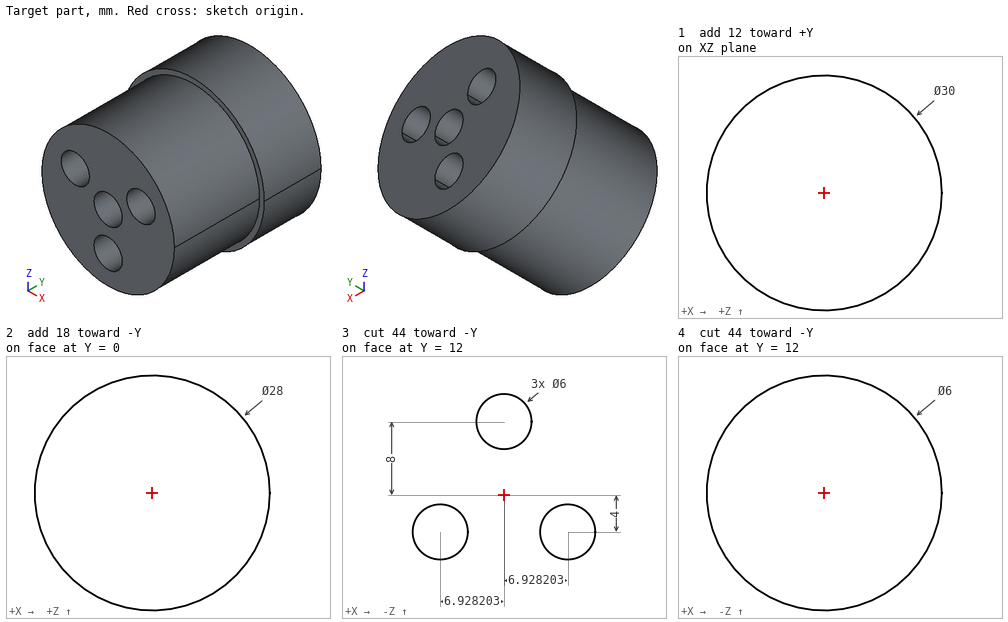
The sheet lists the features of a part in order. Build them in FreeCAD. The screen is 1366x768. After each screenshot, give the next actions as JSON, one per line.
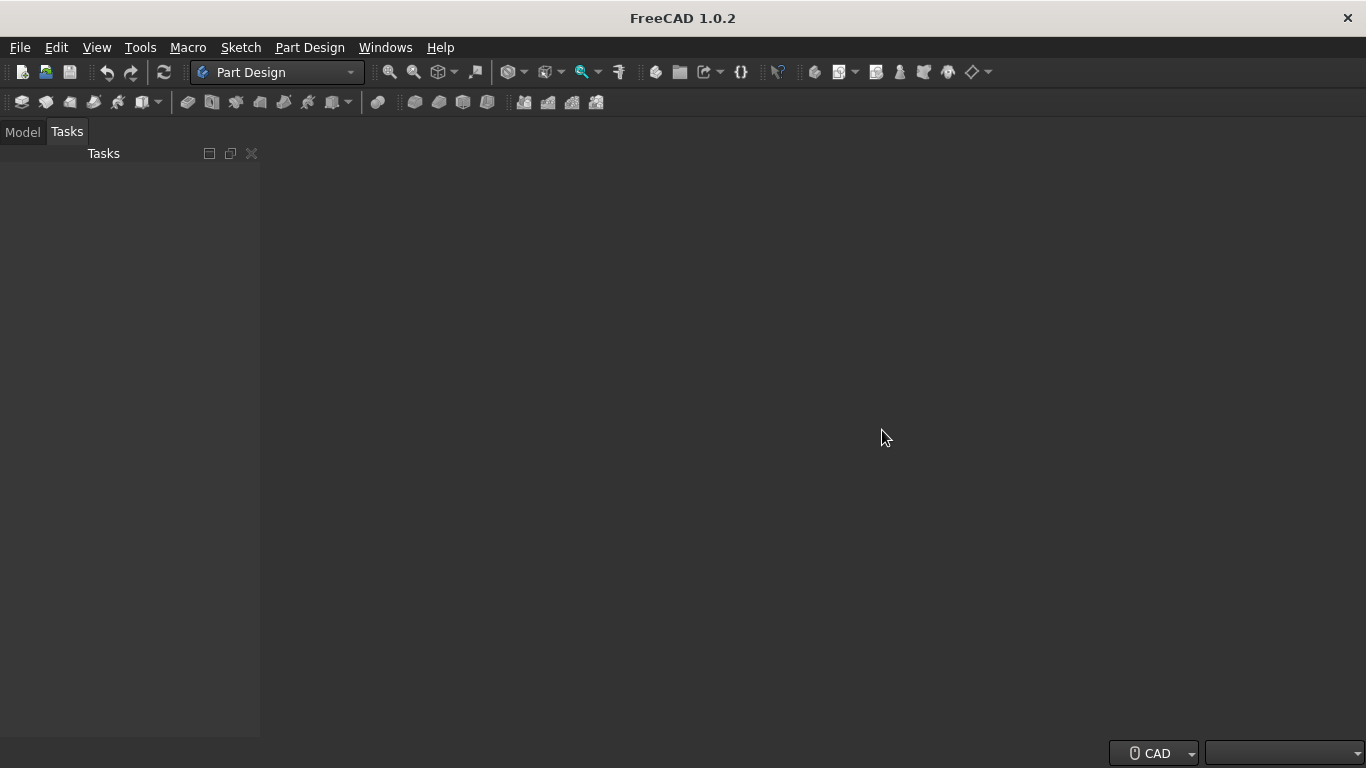
{"action": "left_click", "coordinate": [22, 72]}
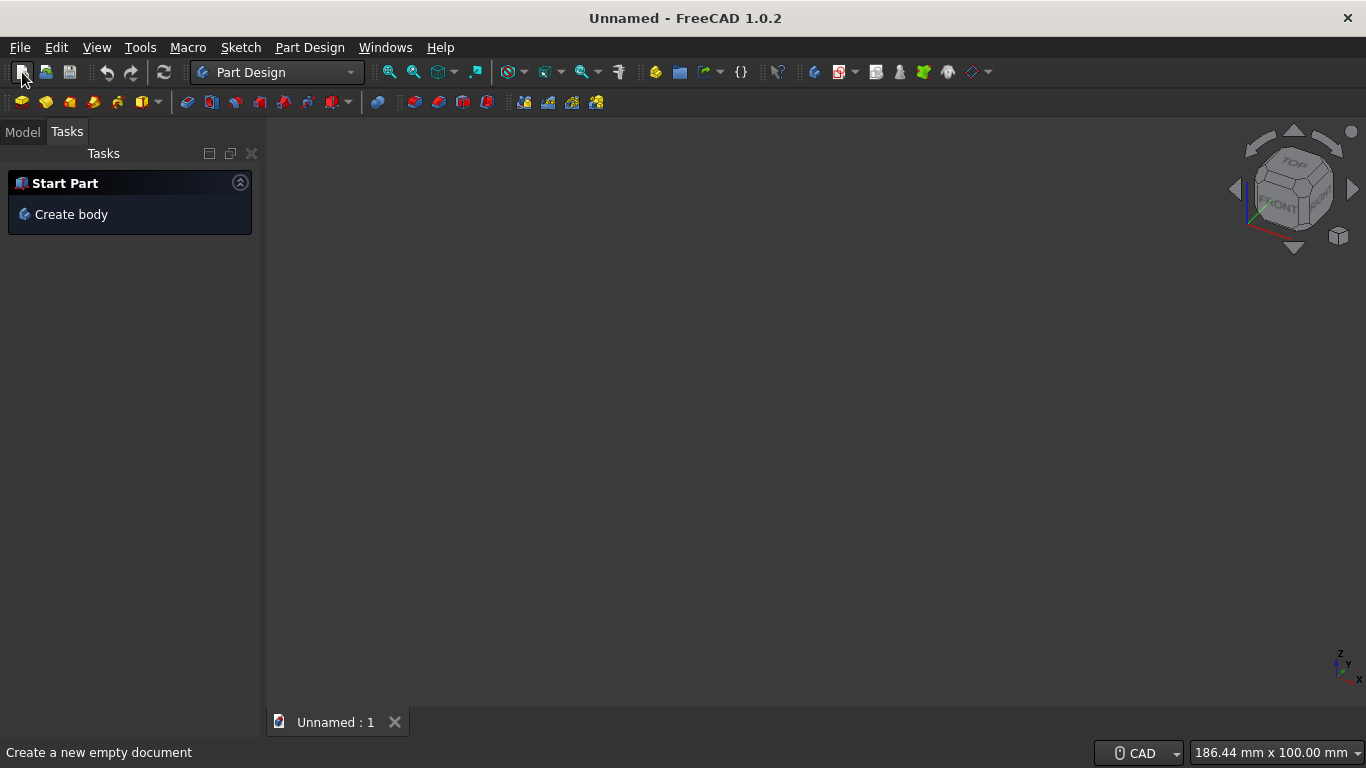
{"action": "left_click", "coordinate": [840, 72]}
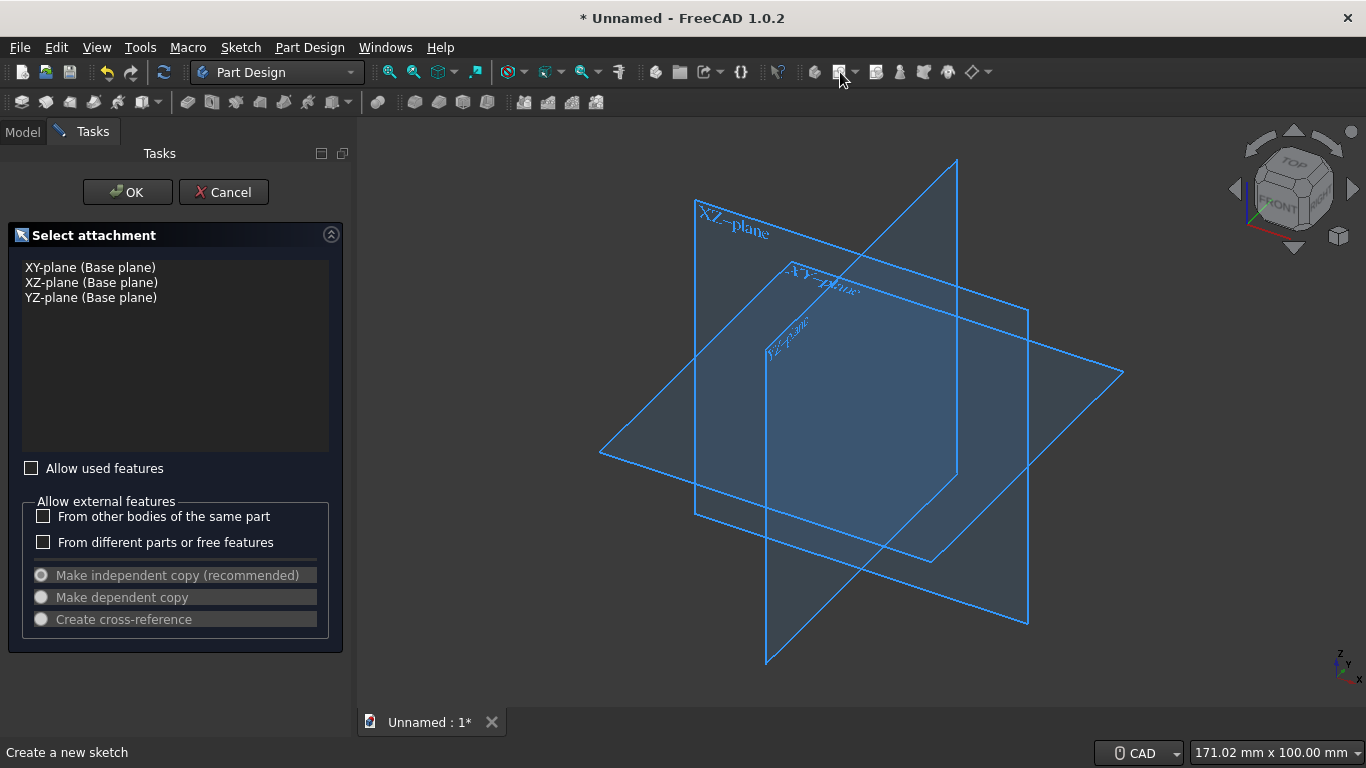
{"action": "left_click", "coordinate": [82, 282]}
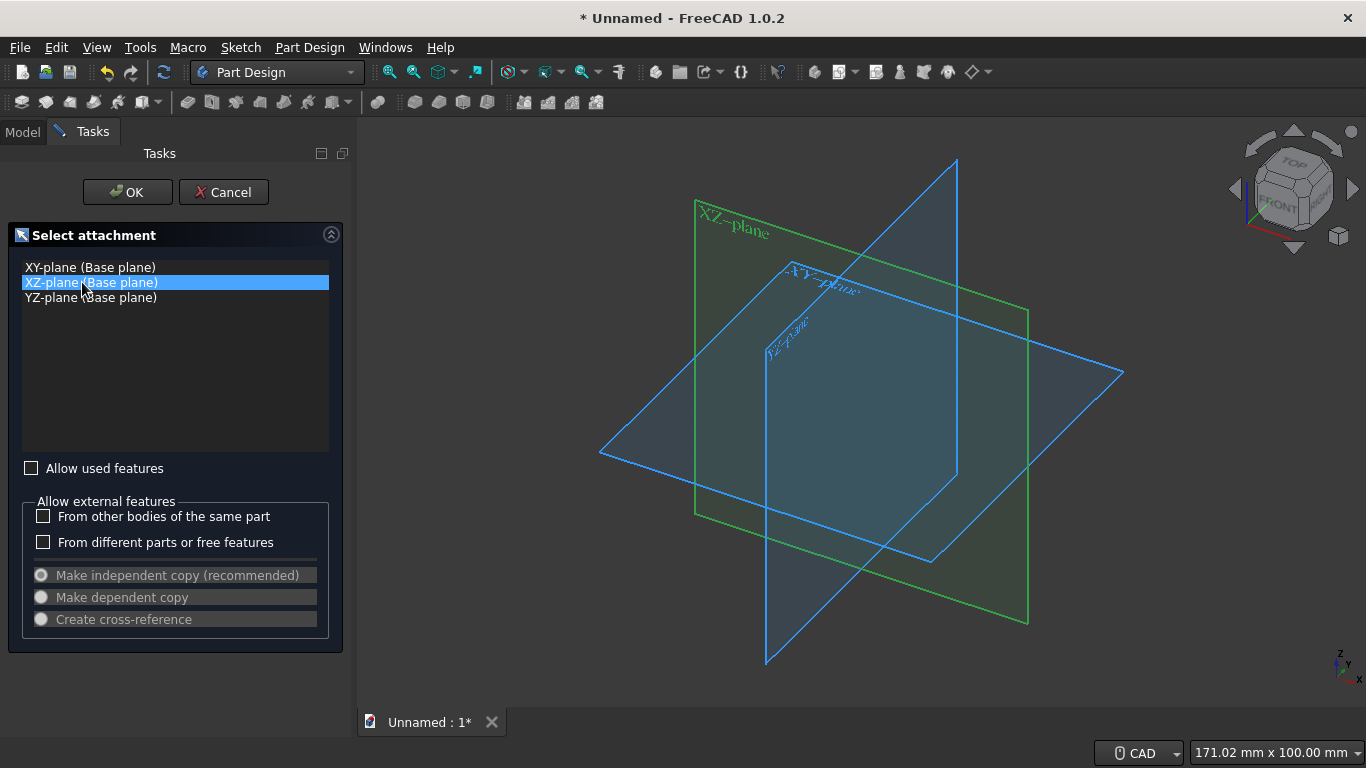
{"action": "left_click", "coordinate": [128, 192]}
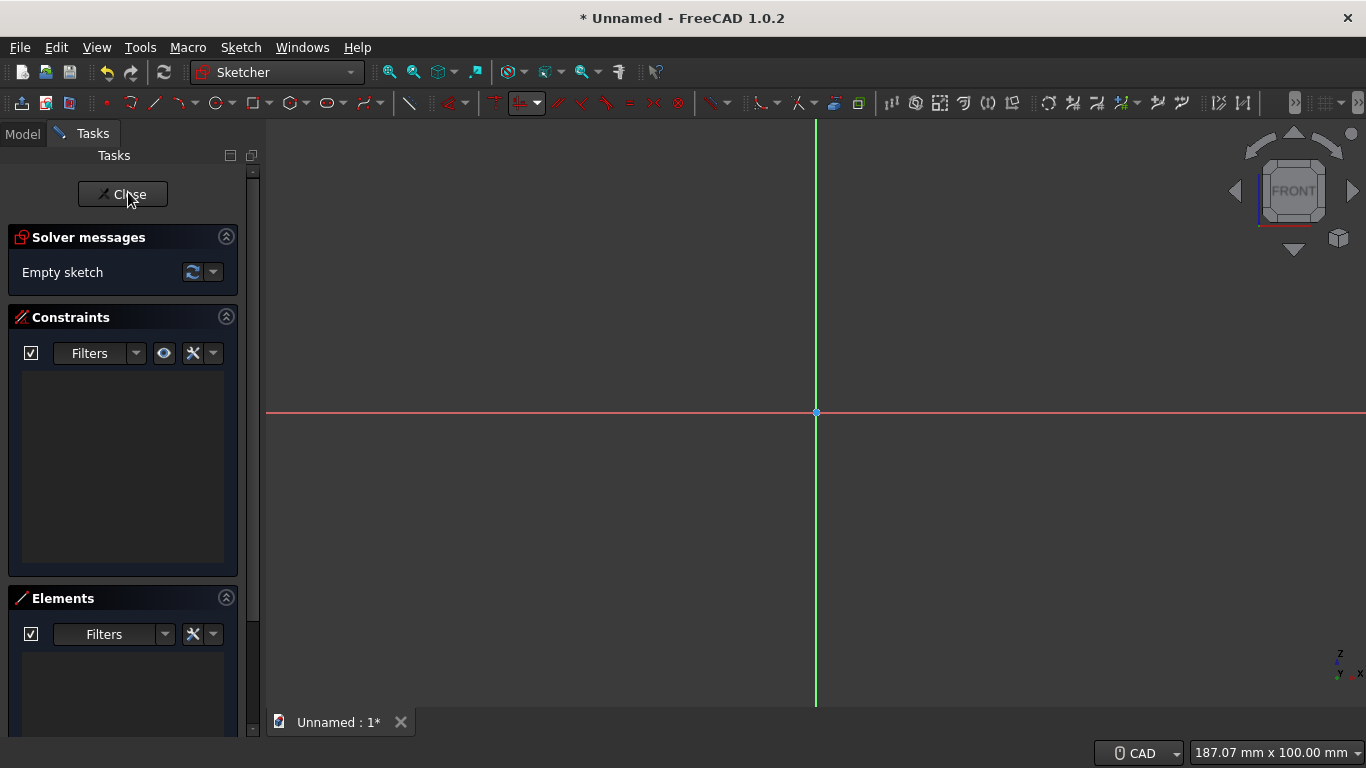
{"action": "scroll", "coordinate": [872, 413], "scroll_direction": "up", "scroll_amount": 4}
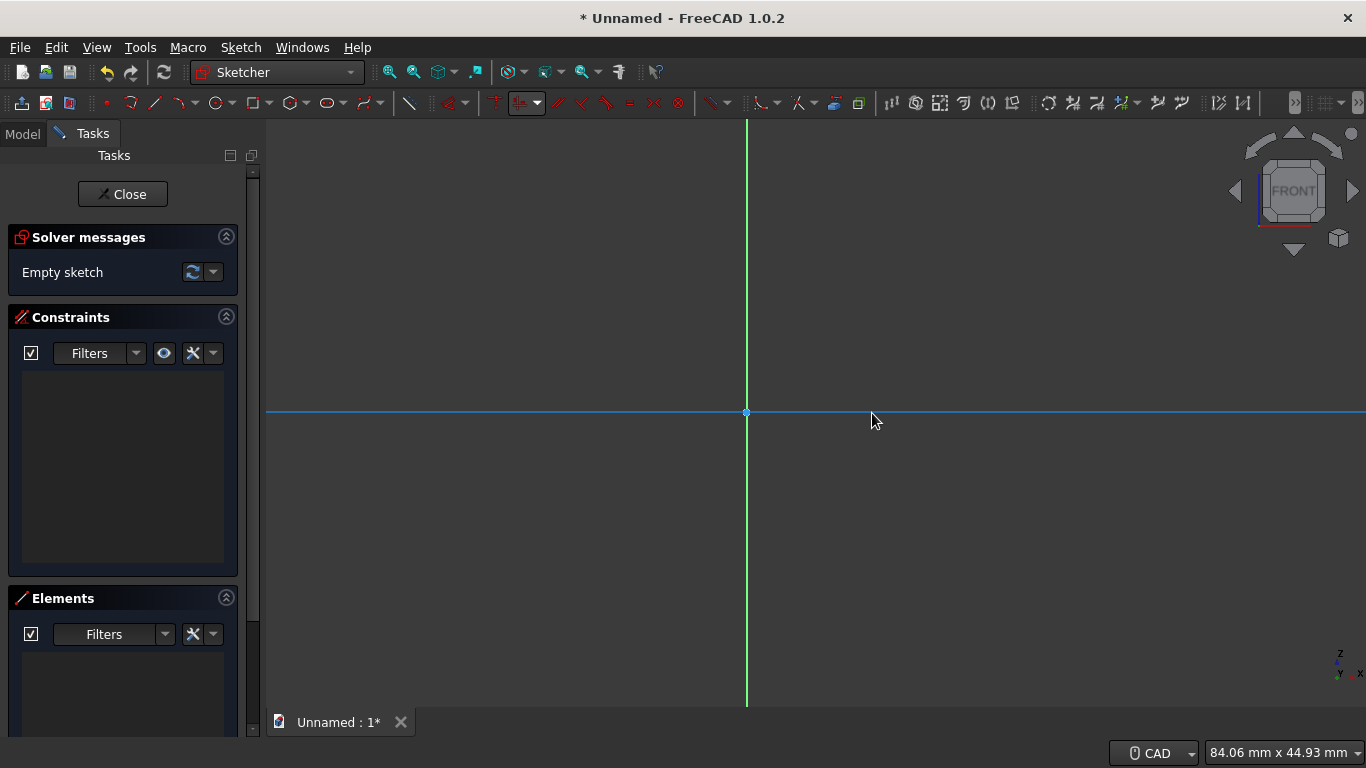
{"action": "left_click", "coordinate": [216, 104]}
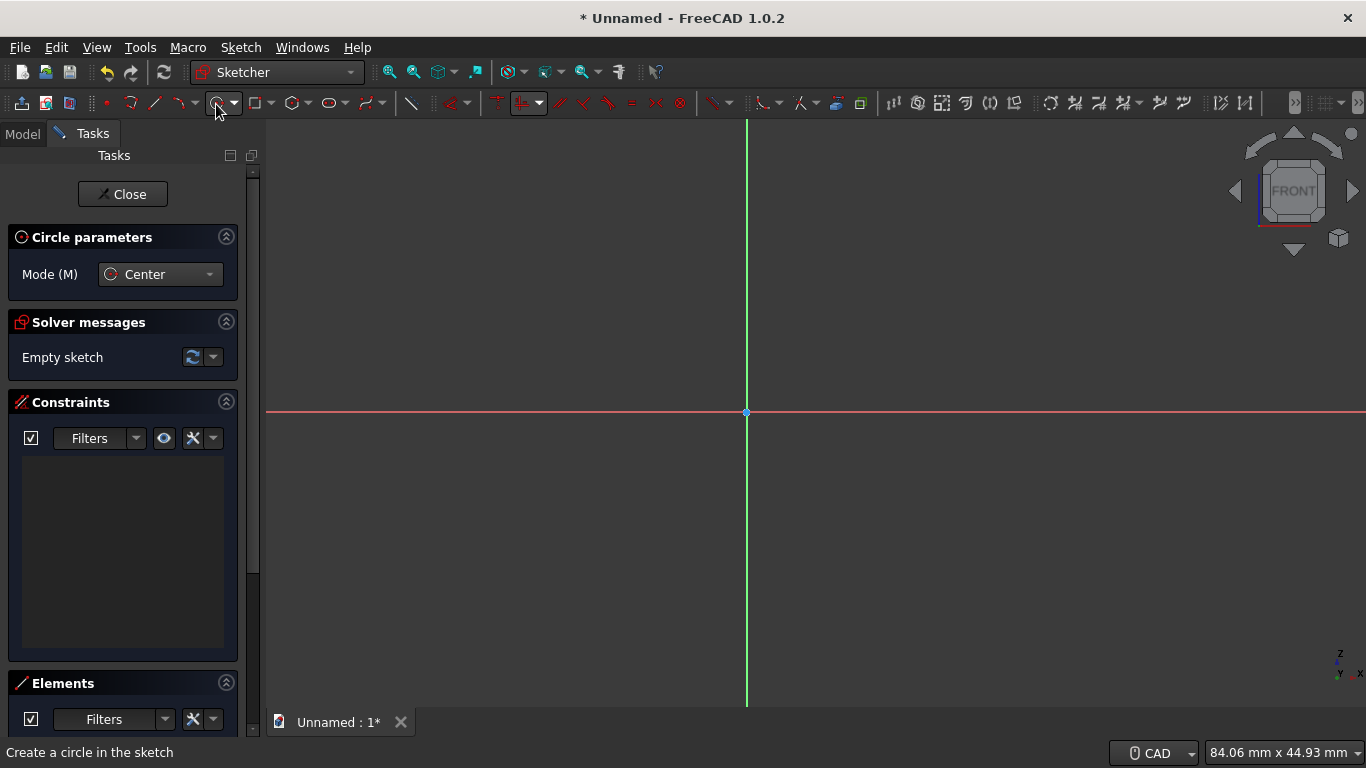
{"action": "left_click", "coordinate": [747, 412]}
{"action": "left_click", "coordinate": [885, 274]}
{"action": "key", "text": "Escape"}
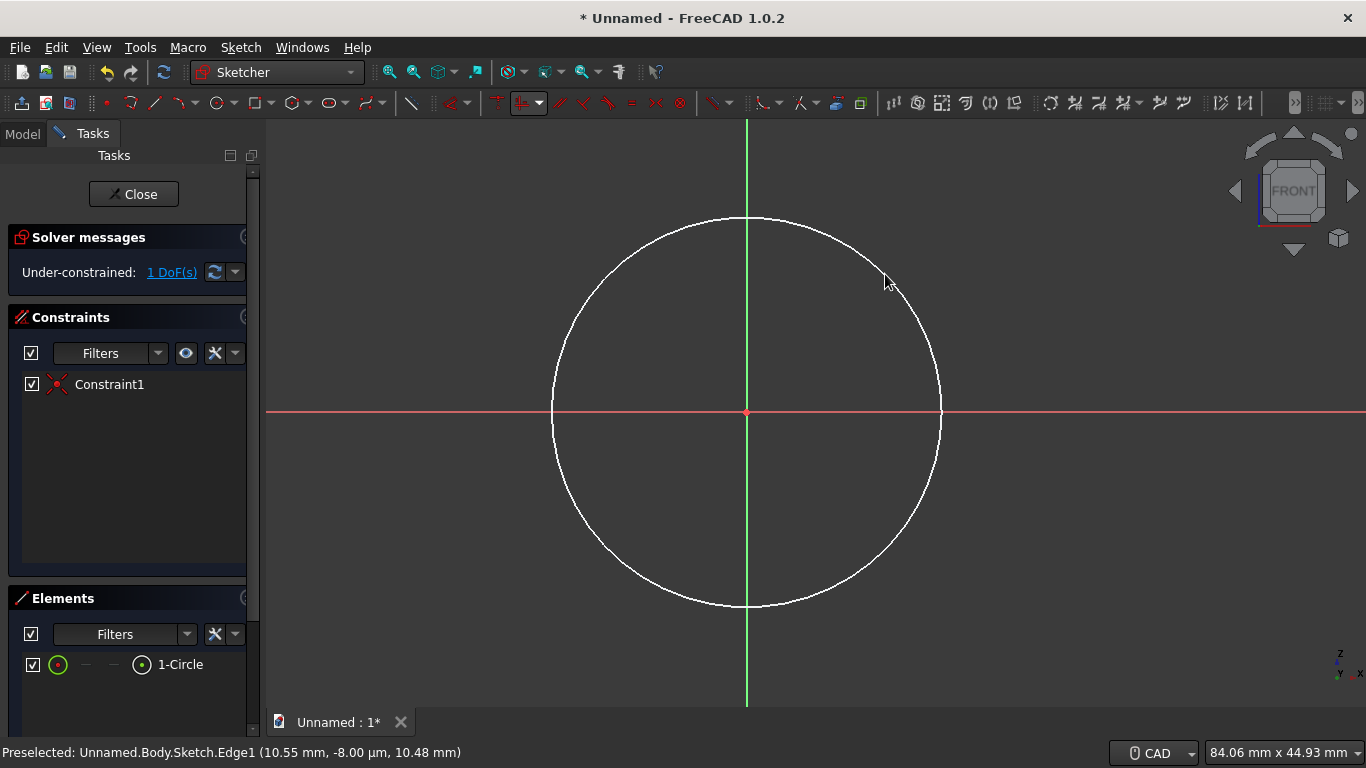
{"action": "left_click", "coordinate": [884, 274]}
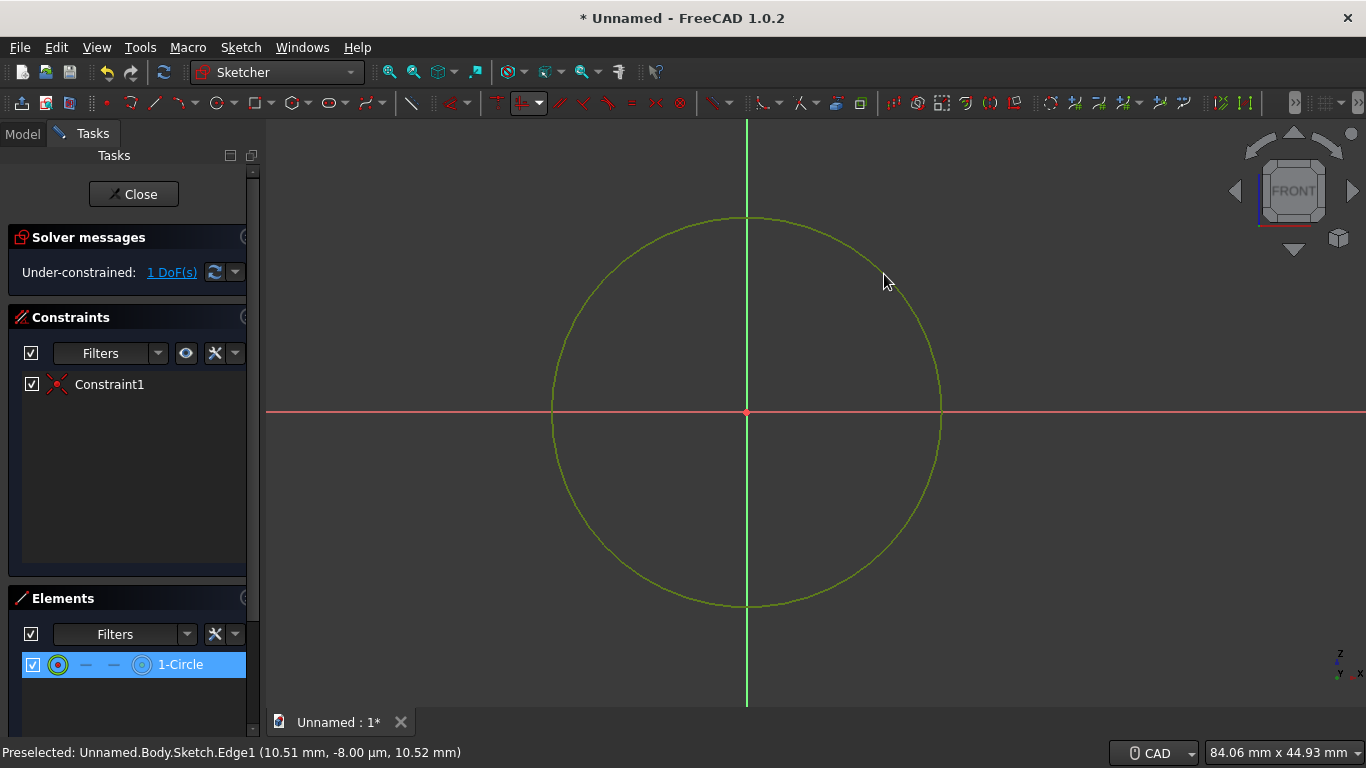
{"action": "left_click", "coordinate": [470, 104]}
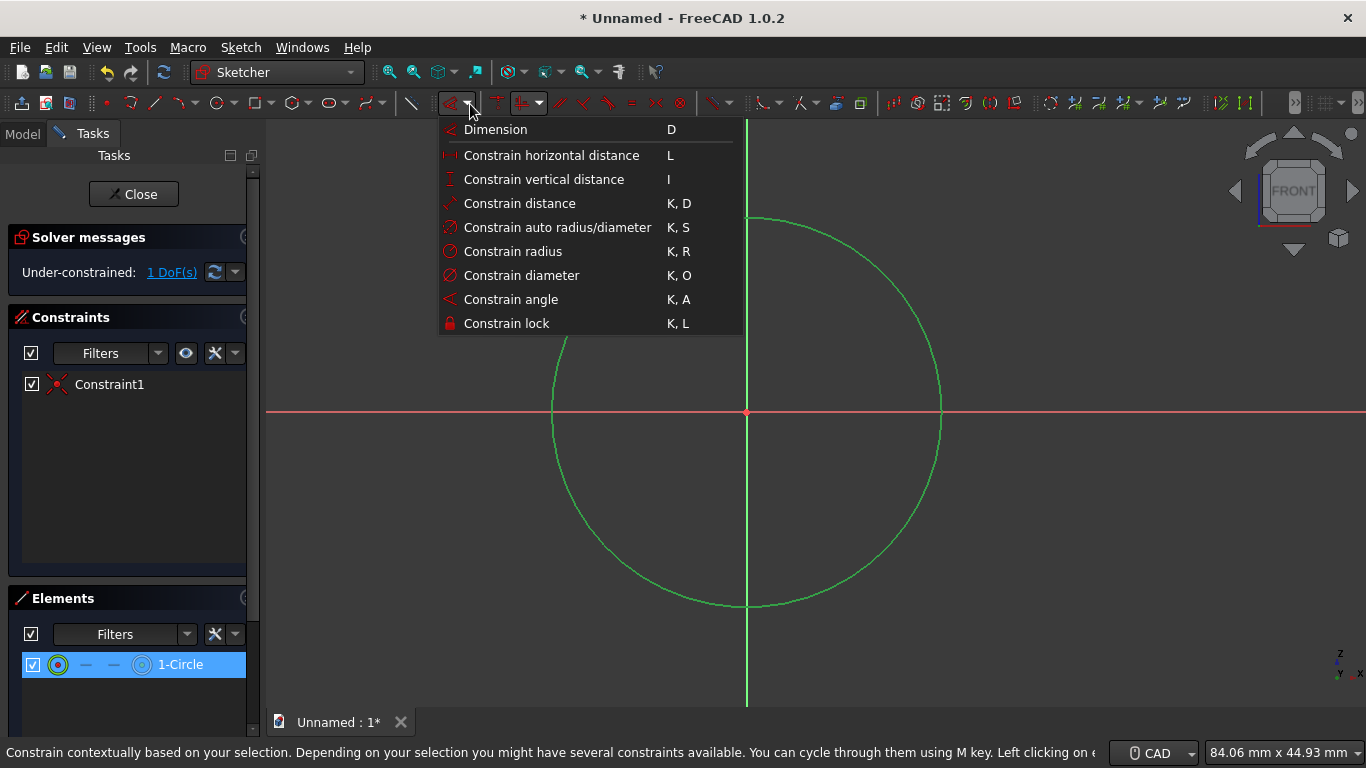
{"action": "left_click", "coordinate": [591, 275]}